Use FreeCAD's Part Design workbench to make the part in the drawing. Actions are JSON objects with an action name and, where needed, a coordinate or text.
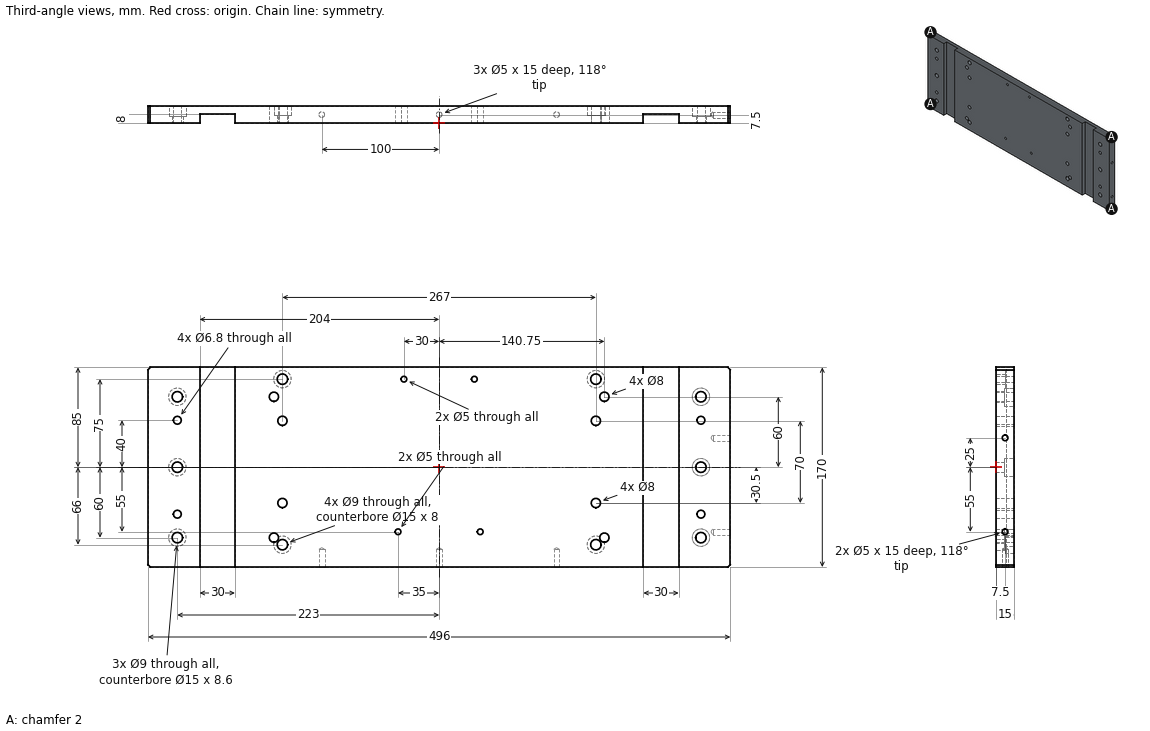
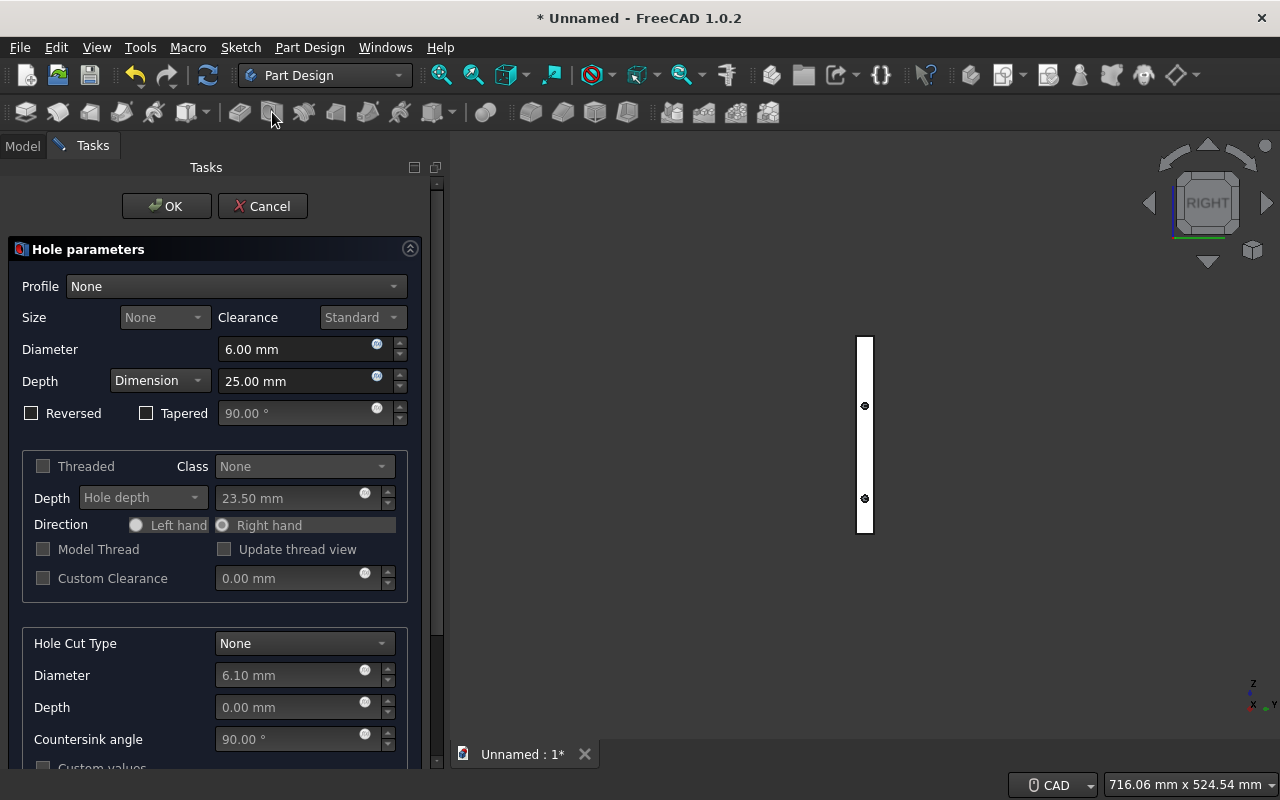
{"action": "triple_click", "coordinate": [305, 349]}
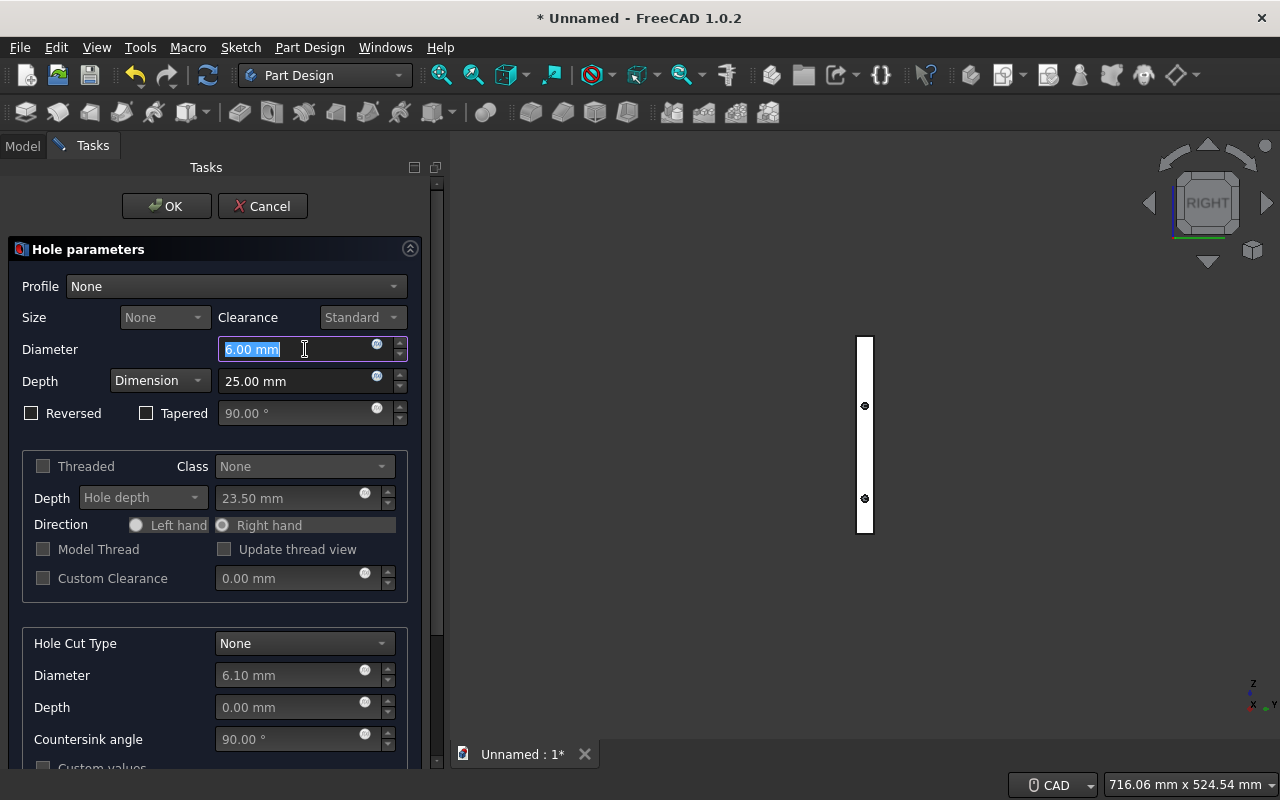
{"action": "type", "text": "5"}
{"action": "key", "text": "Tab"}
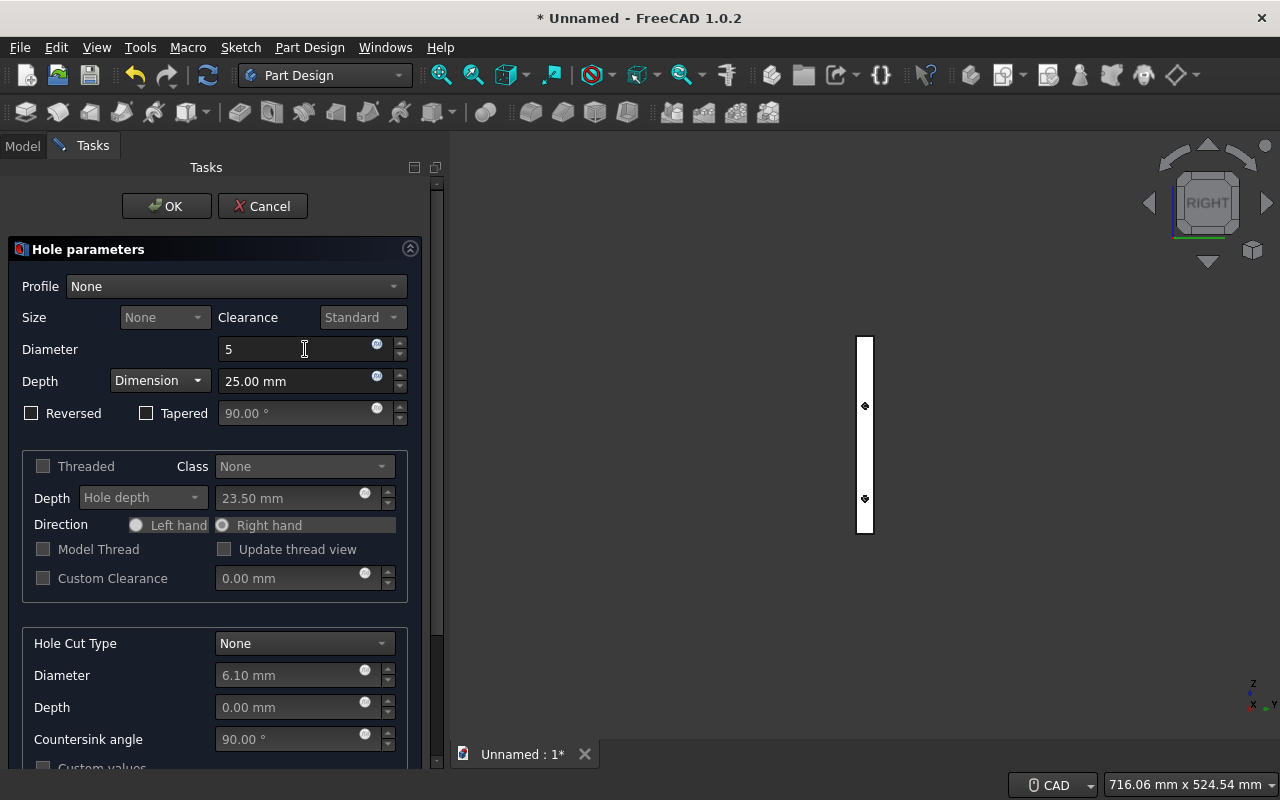
{"action": "triple_click", "coordinate": [305, 381]}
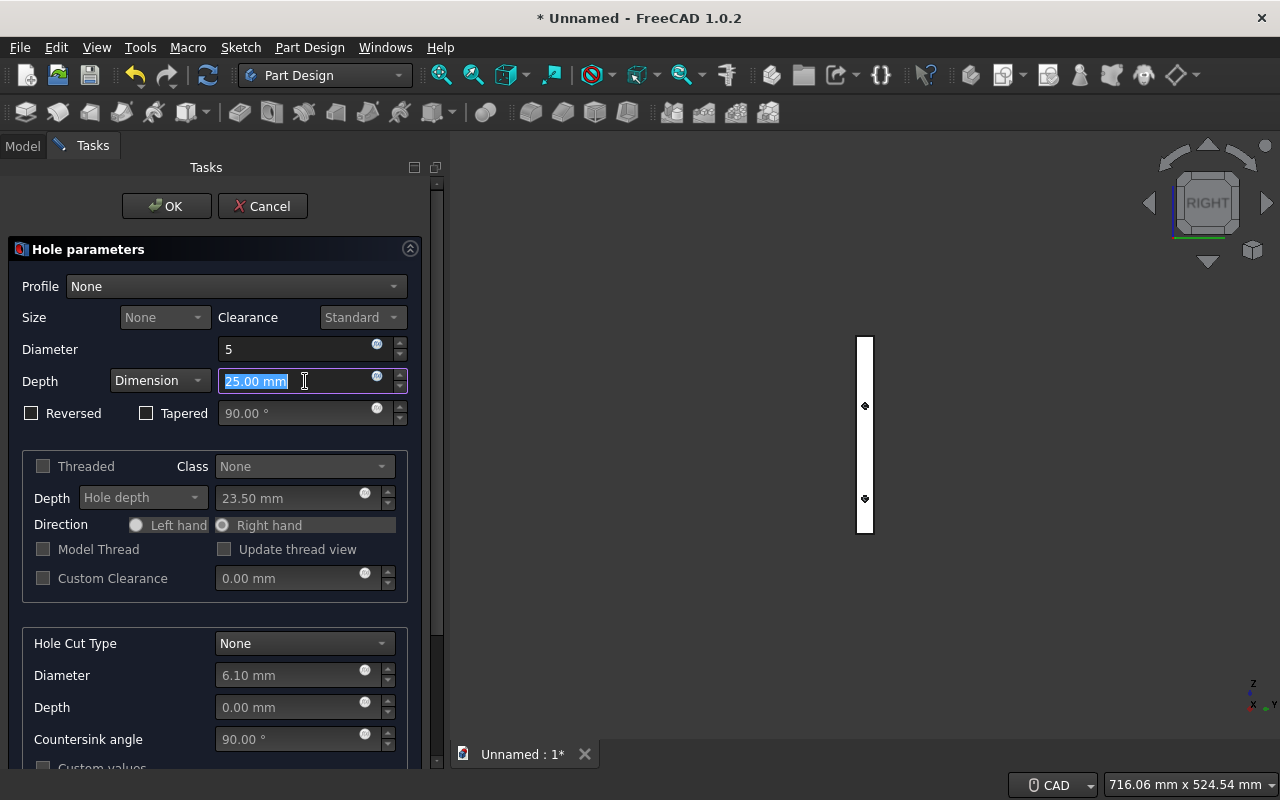
{"action": "type", "text": "15"}
{"action": "key", "text": "Tab"}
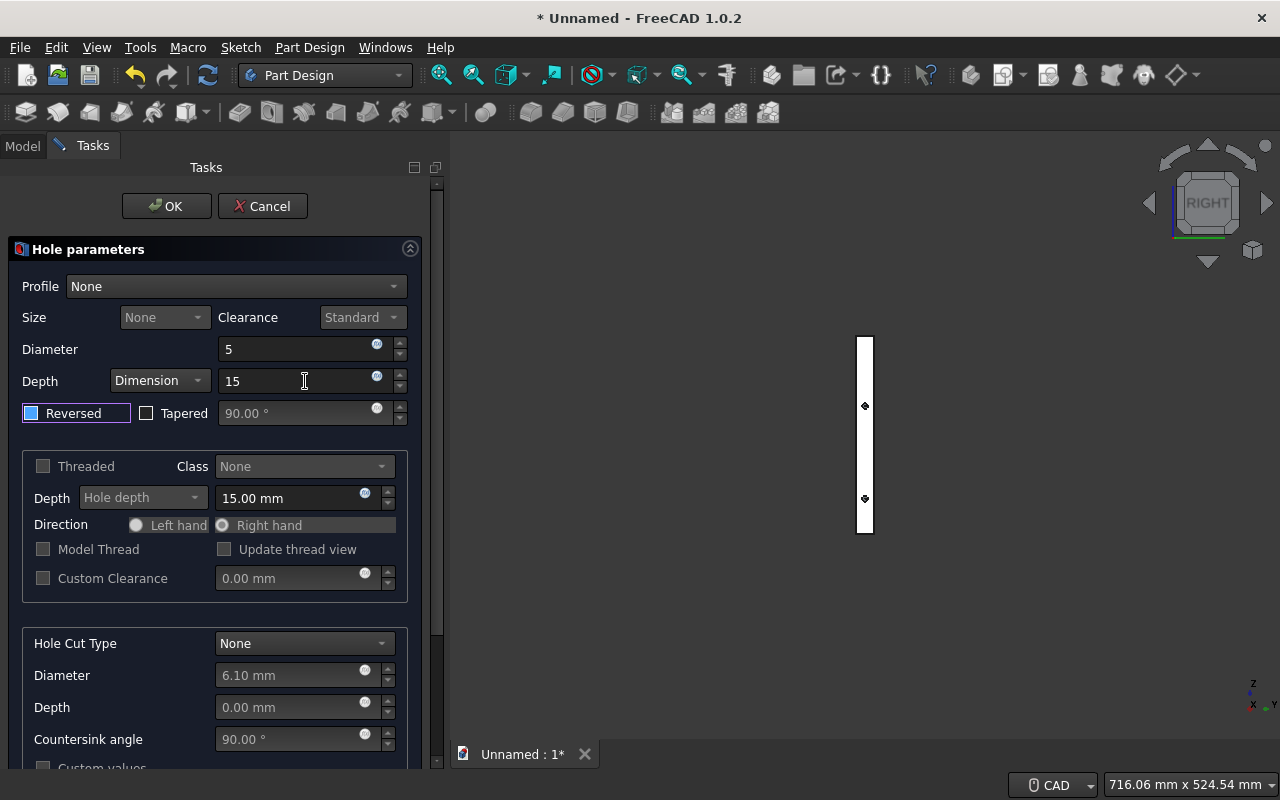
{"action": "left_click", "coordinate": [167, 206]}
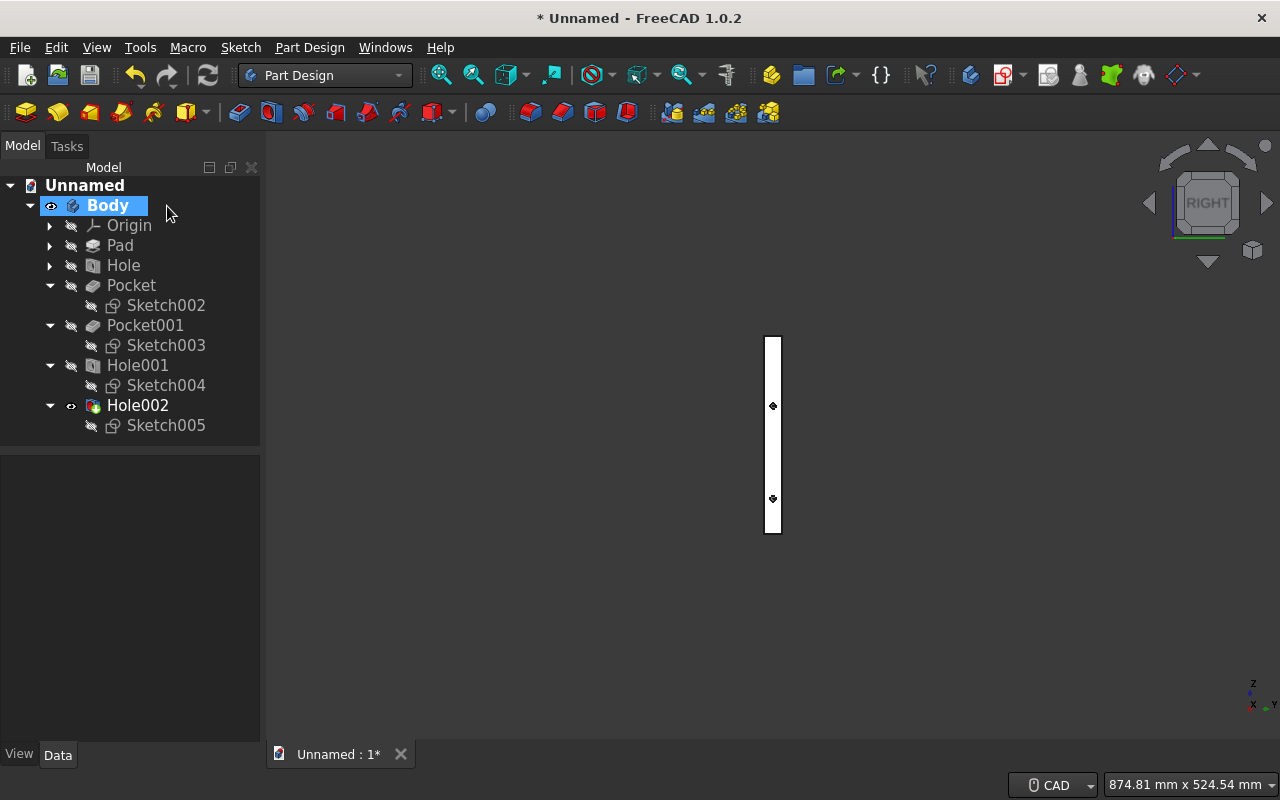
{"action": "left_click", "coordinate": [442, 76]}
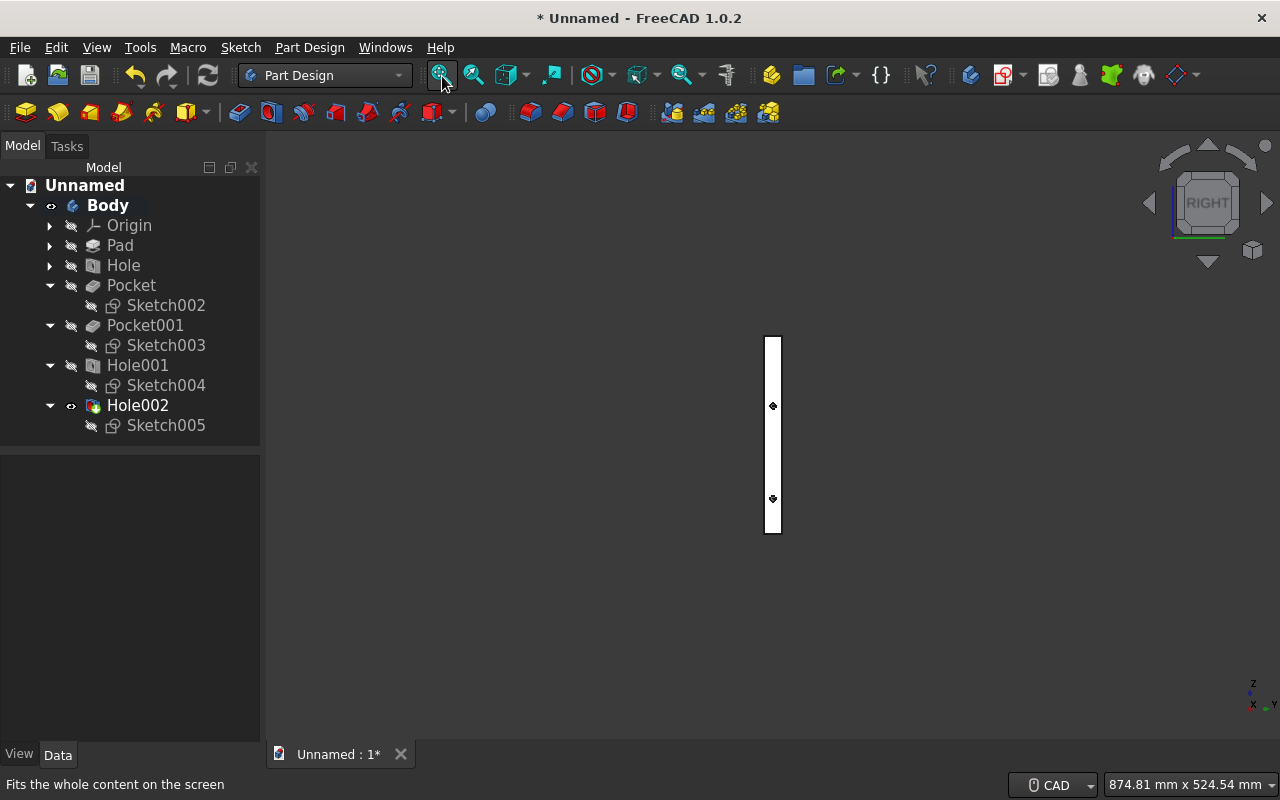
{"action": "left_click", "coordinate": [1004, 76]}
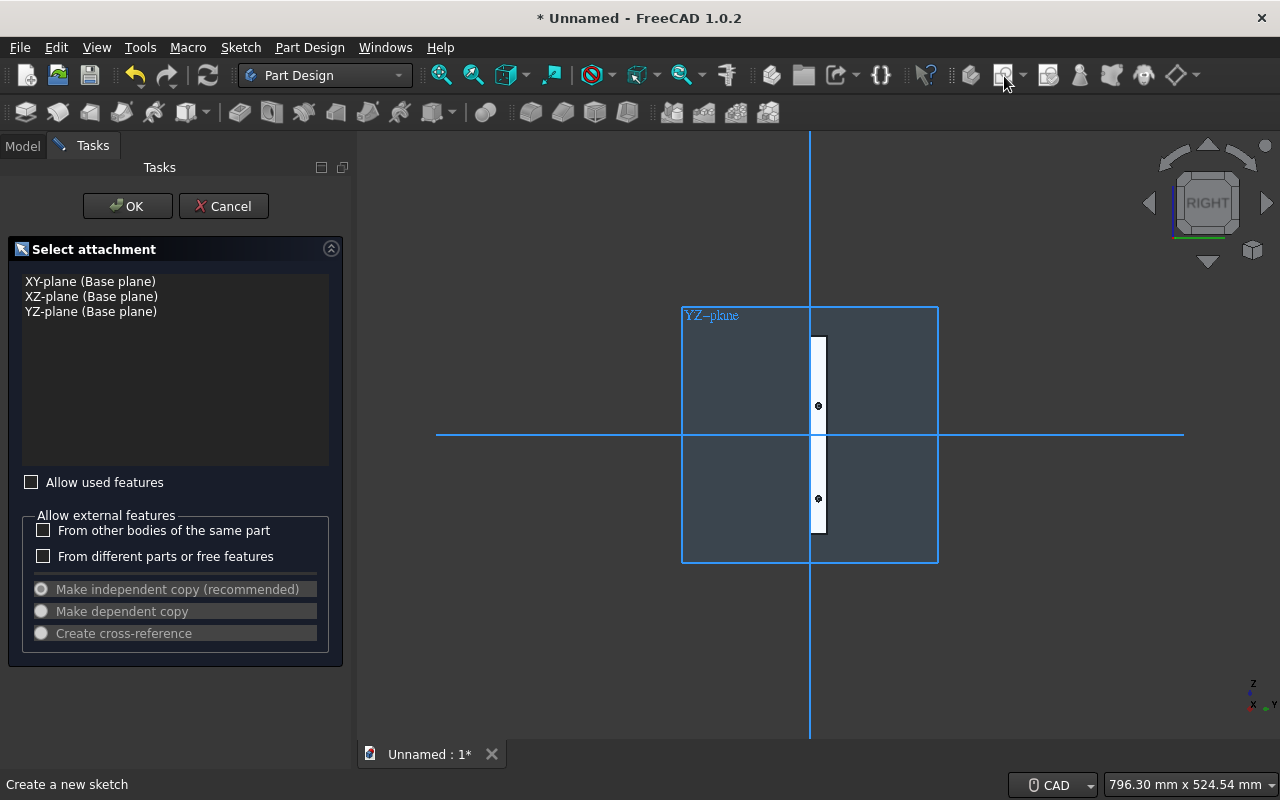
{"action": "left_click", "coordinate": [82, 296]}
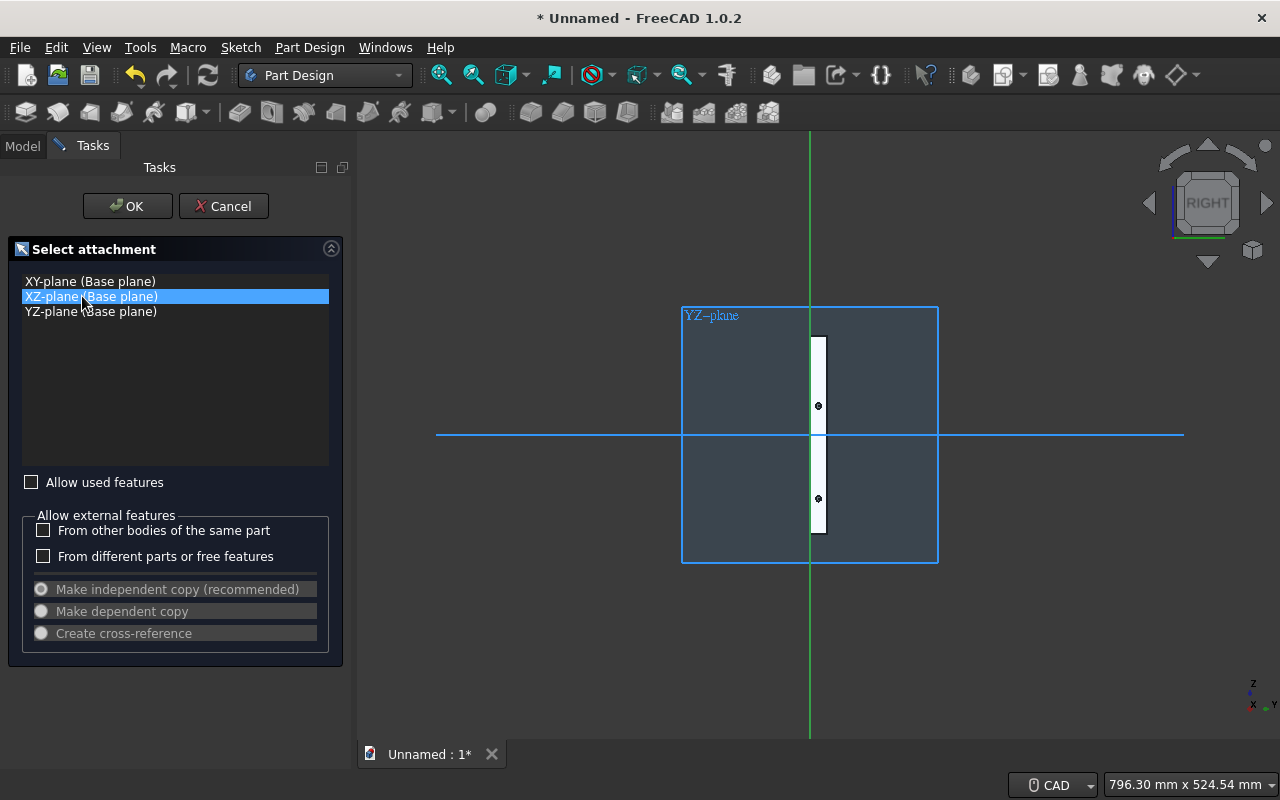
{"action": "left_click", "coordinate": [128, 206]}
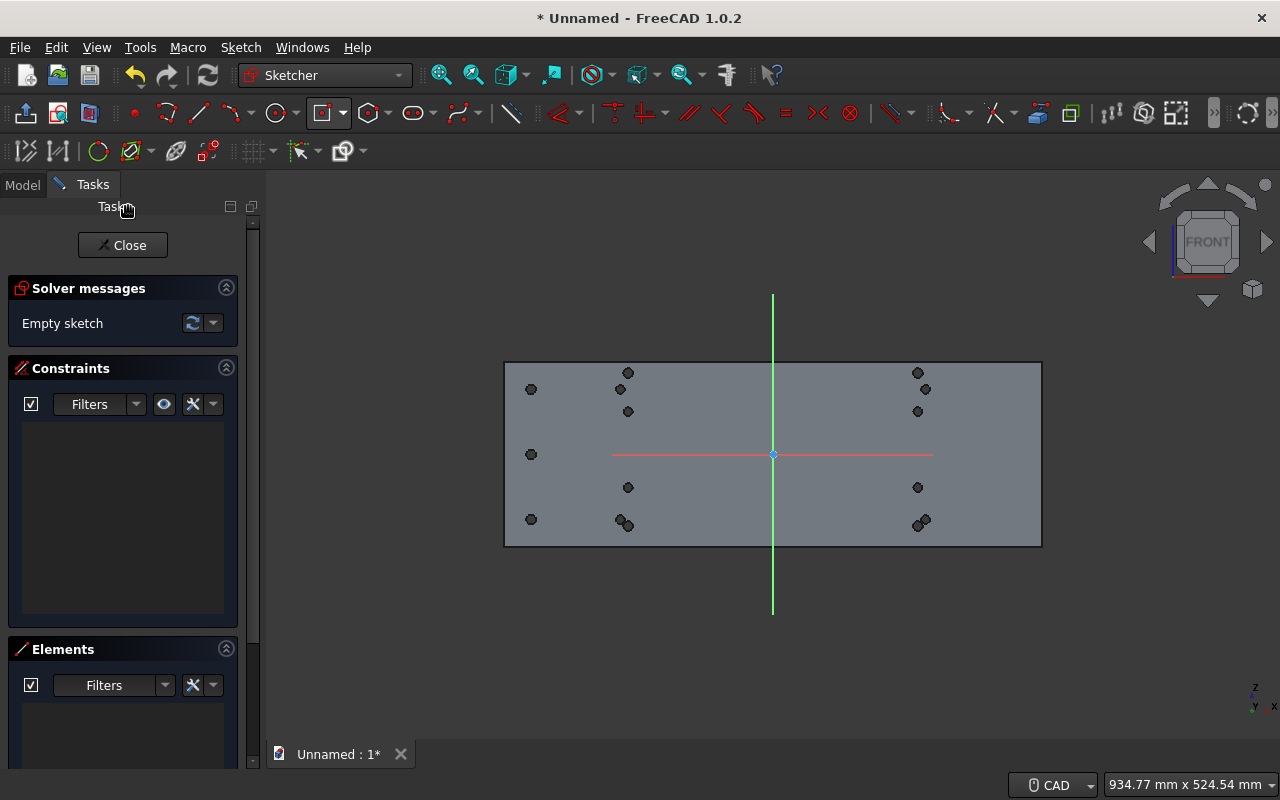
{"action": "scroll", "coordinate": [787, 492], "scroll_direction": "up", "scroll_amount": 9}